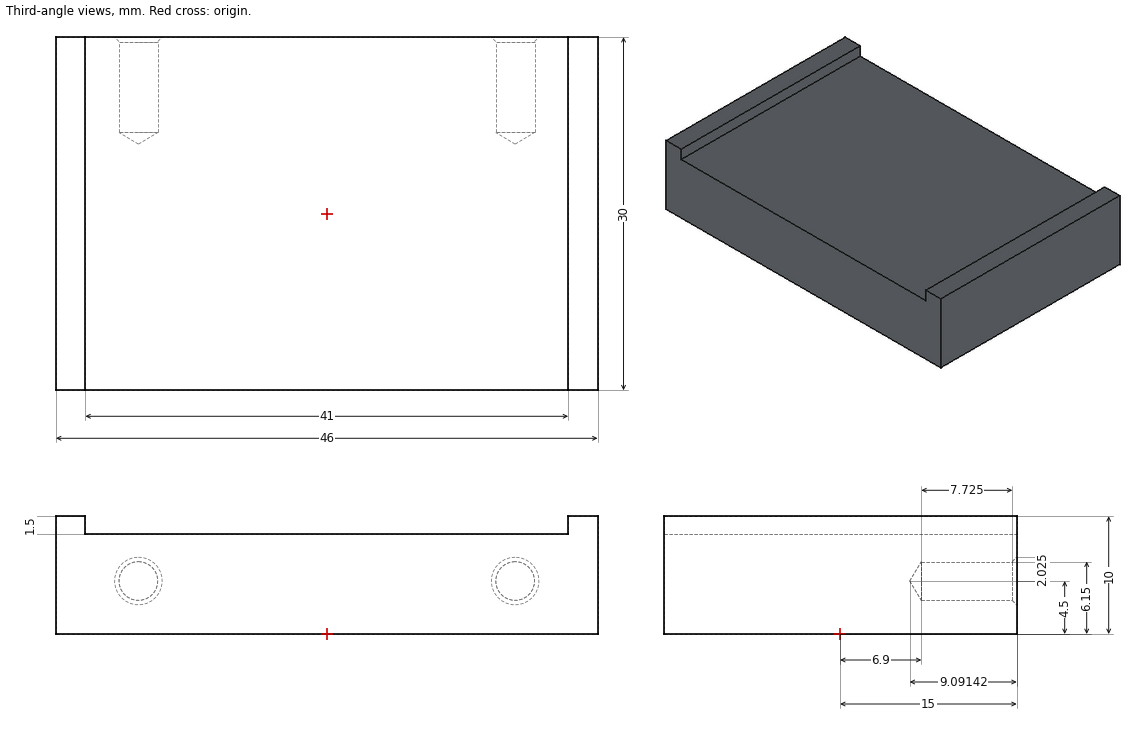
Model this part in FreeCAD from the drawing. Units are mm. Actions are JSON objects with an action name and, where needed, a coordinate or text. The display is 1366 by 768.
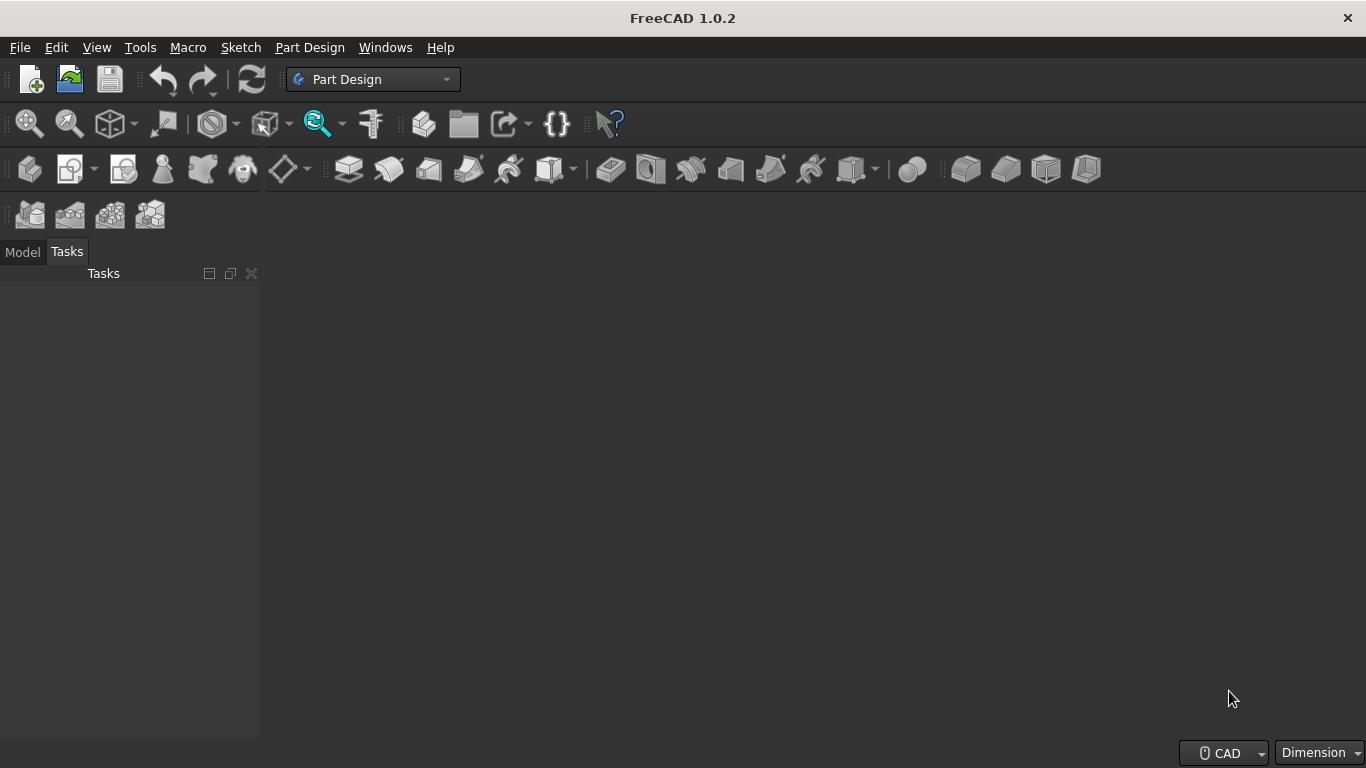
{"action": "left_click", "coordinate": [30, 80]}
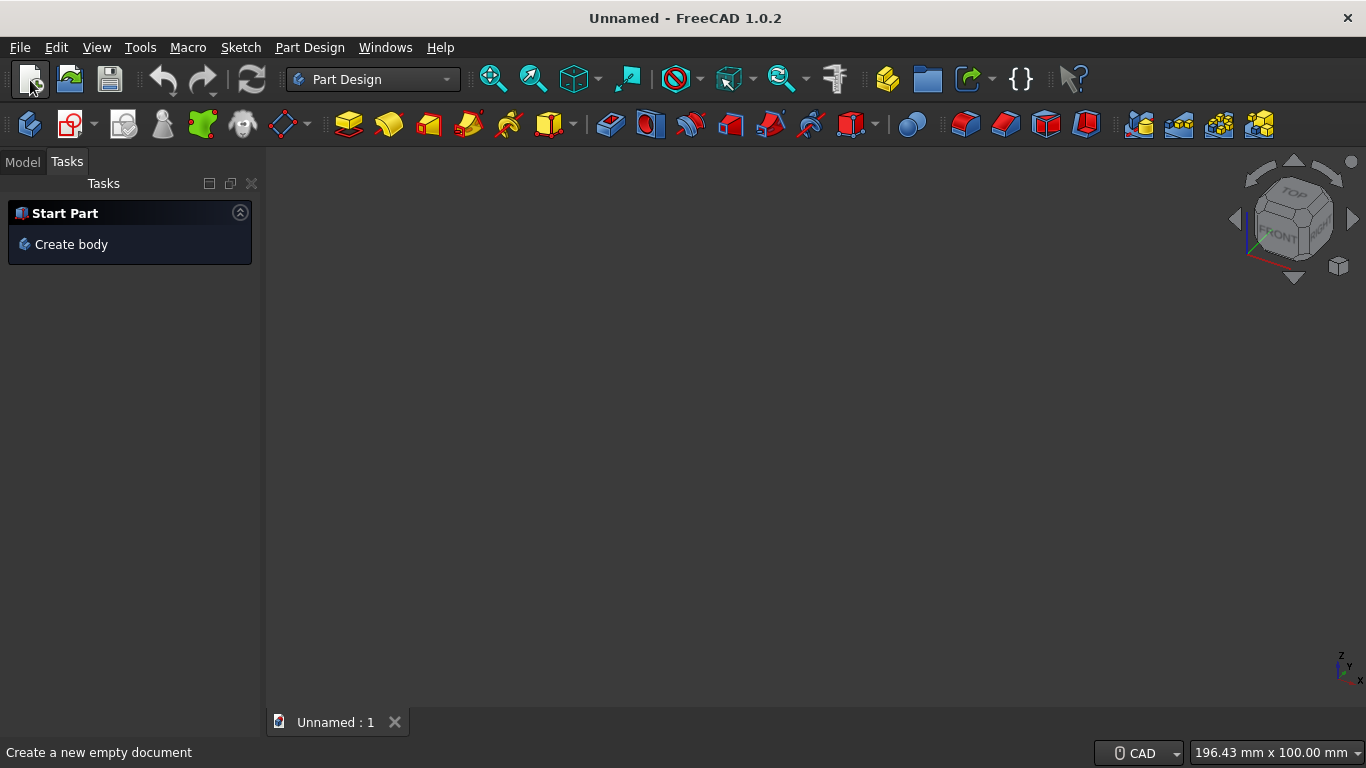
{"action": "left_click", "coordinate": [70, 124]}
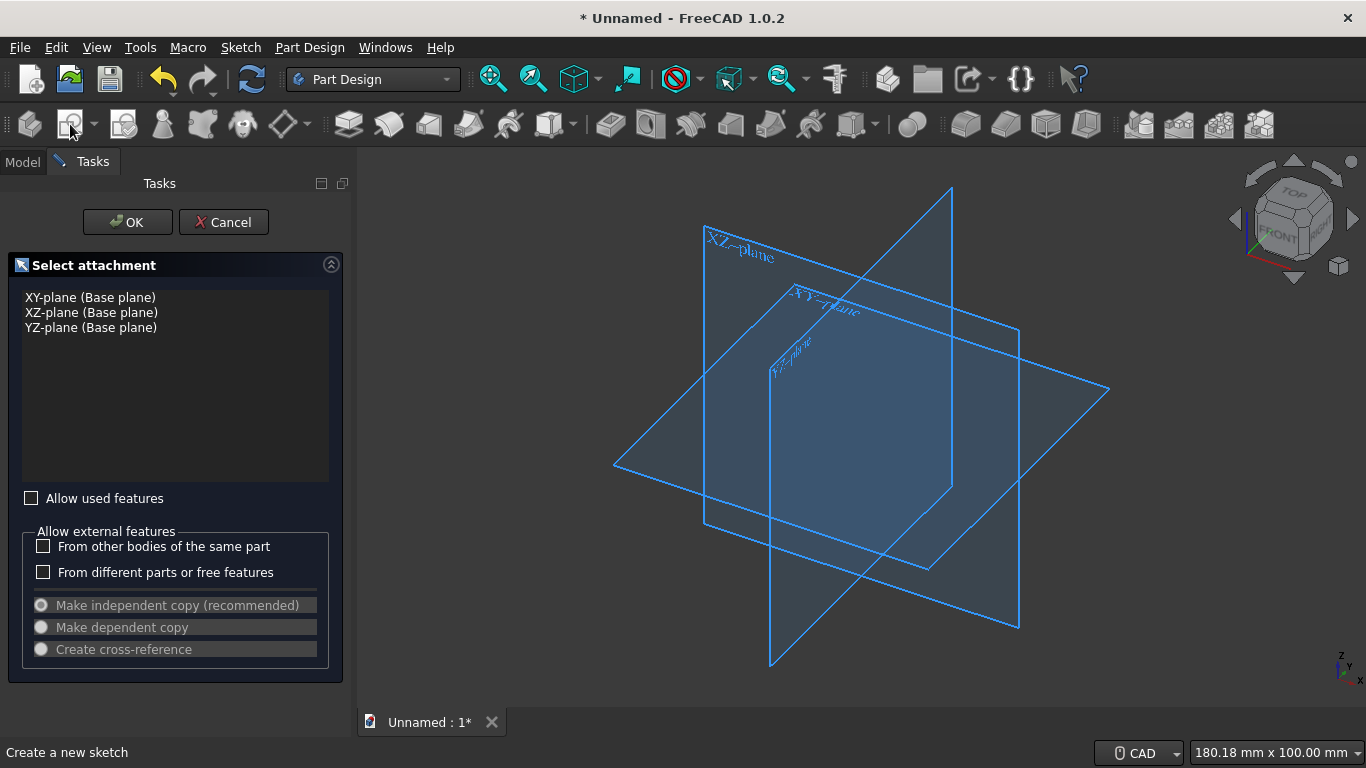
{"action": "left_click", "coordinate": [82, 298]}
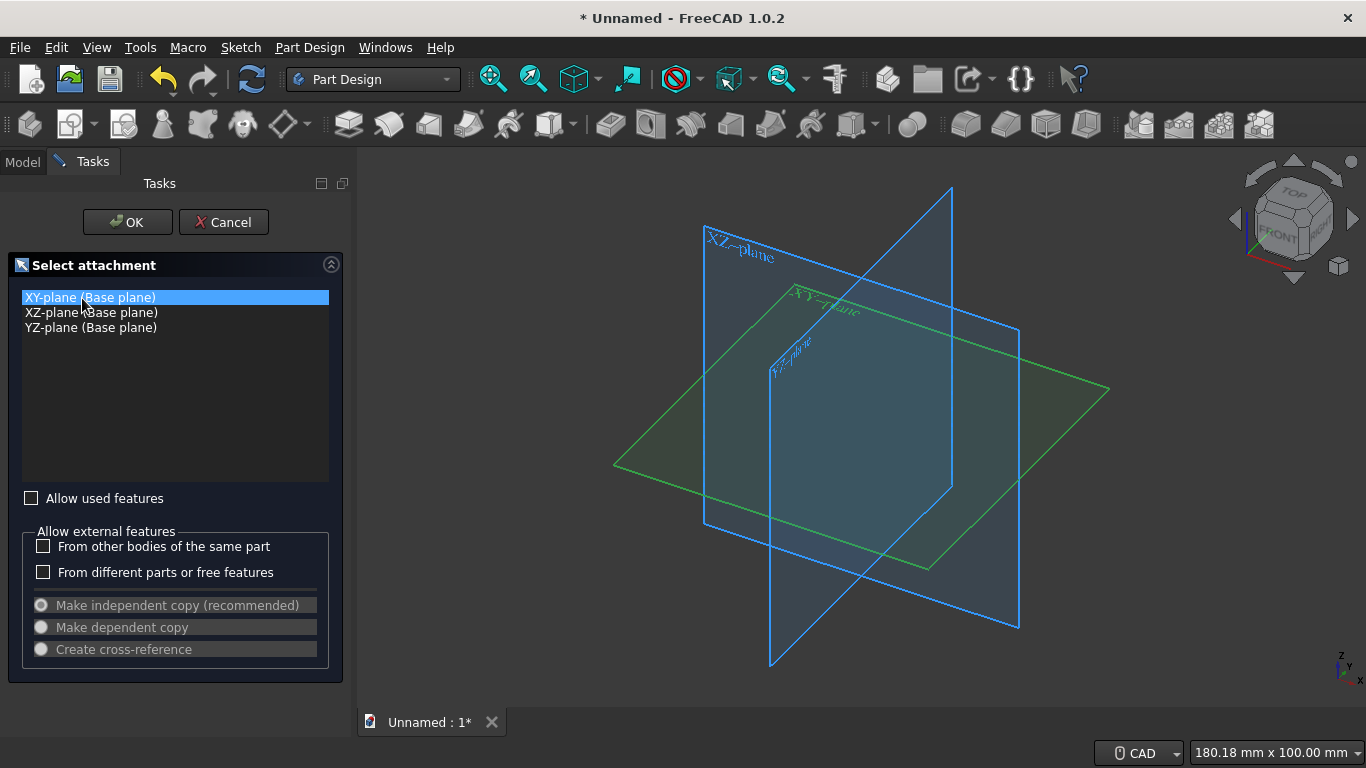
{"action": "left_click", "coordinate": [128, 222]}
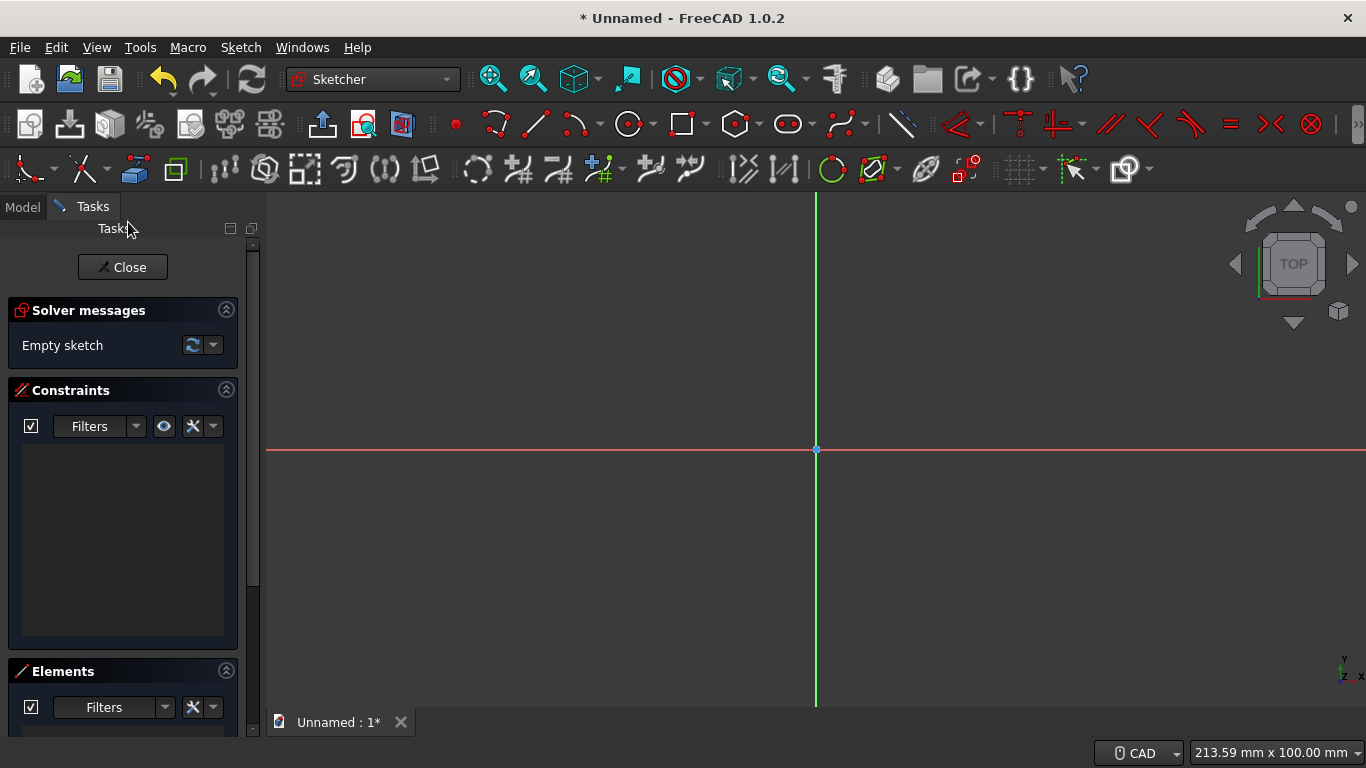
{"action": "scroll", "coordinate": [872, 450], "scroll_direction": "up", "scroll_amount": 4}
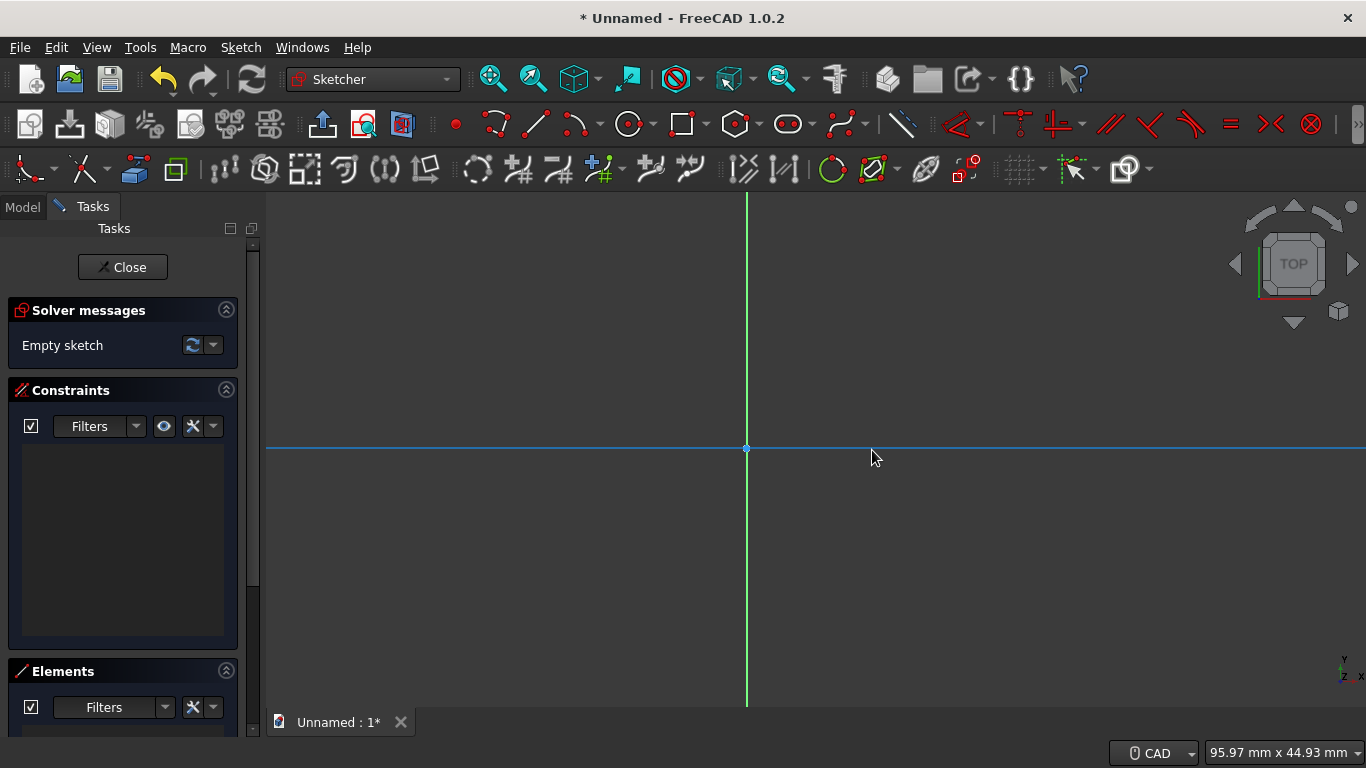
{"action": "left_click", "coordinate": [708, 124]}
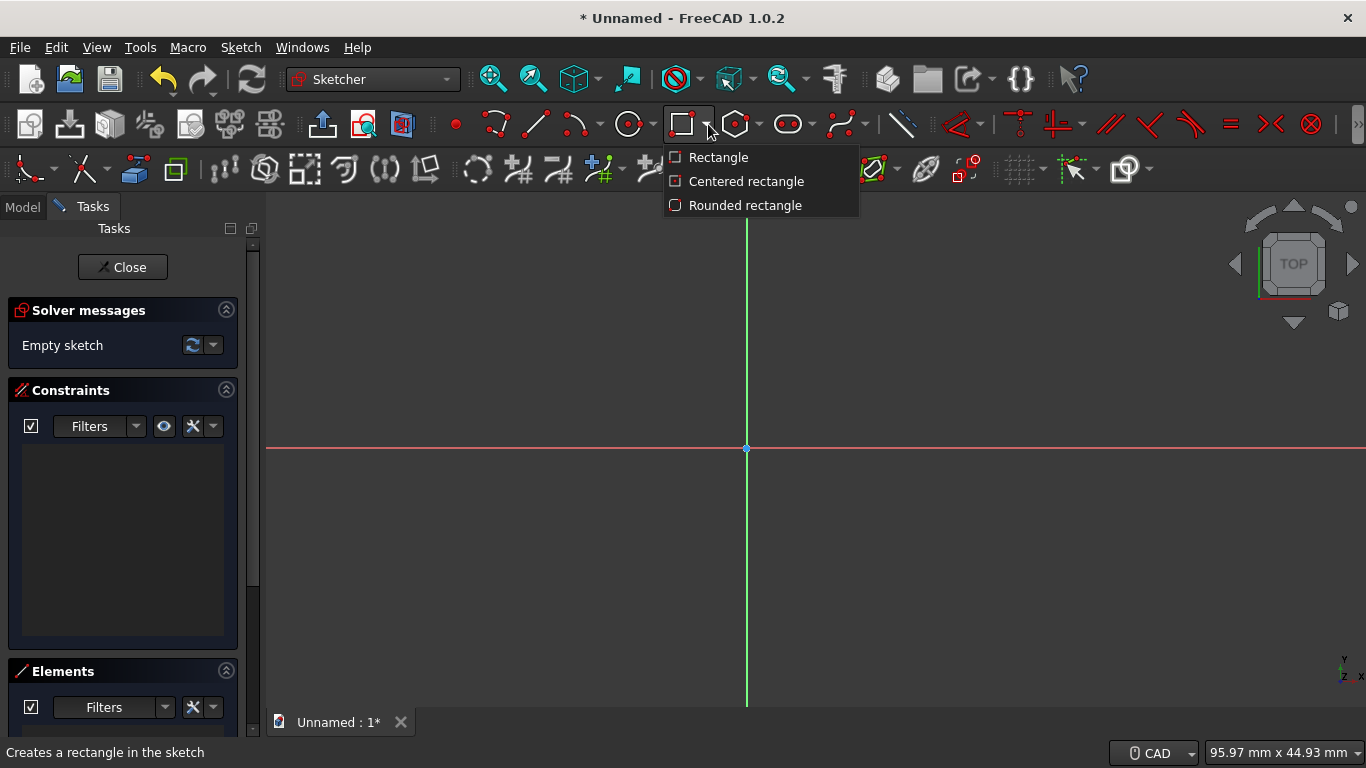
{"action": "left_click", "coordinate": [762, 181]}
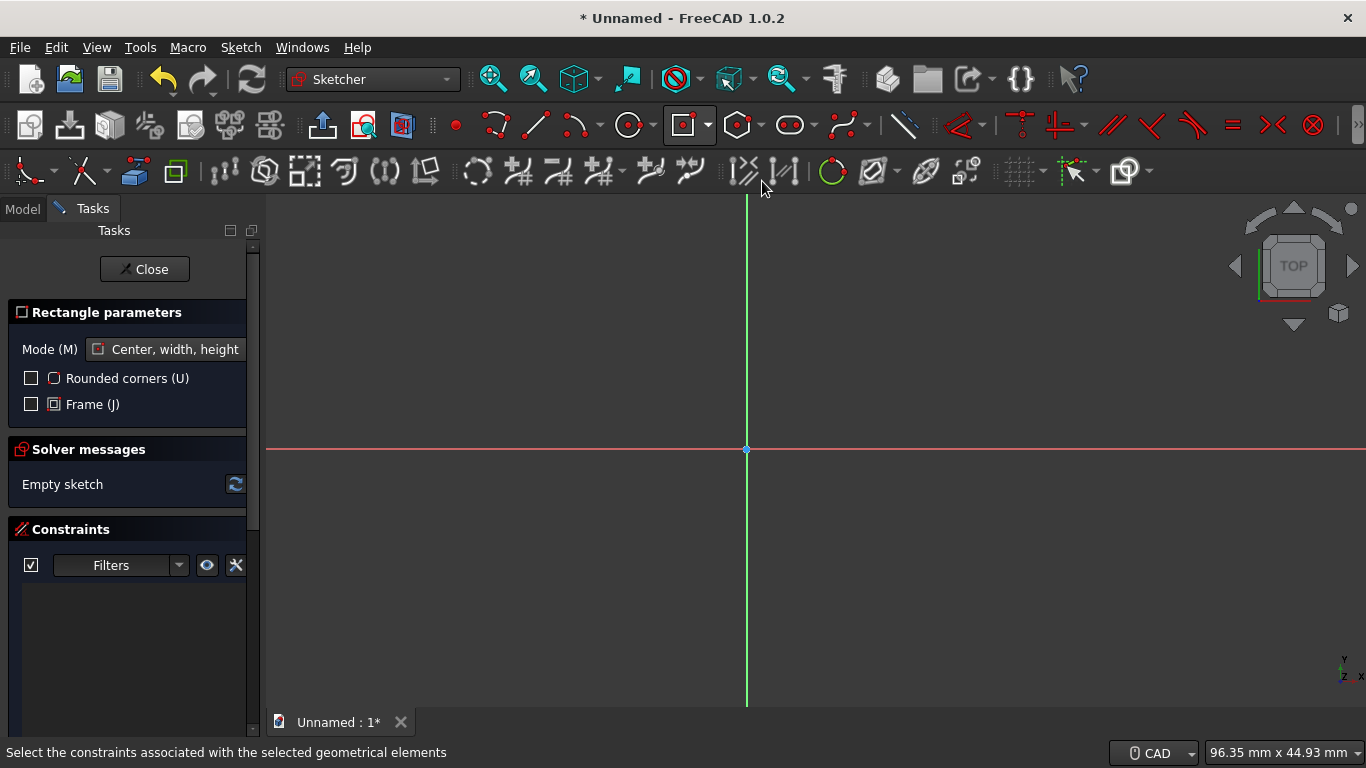
{"action": "left_click", "coordinate": [747, 449]}
{"action": "mouse_move", "coordinate": [1010, 278]}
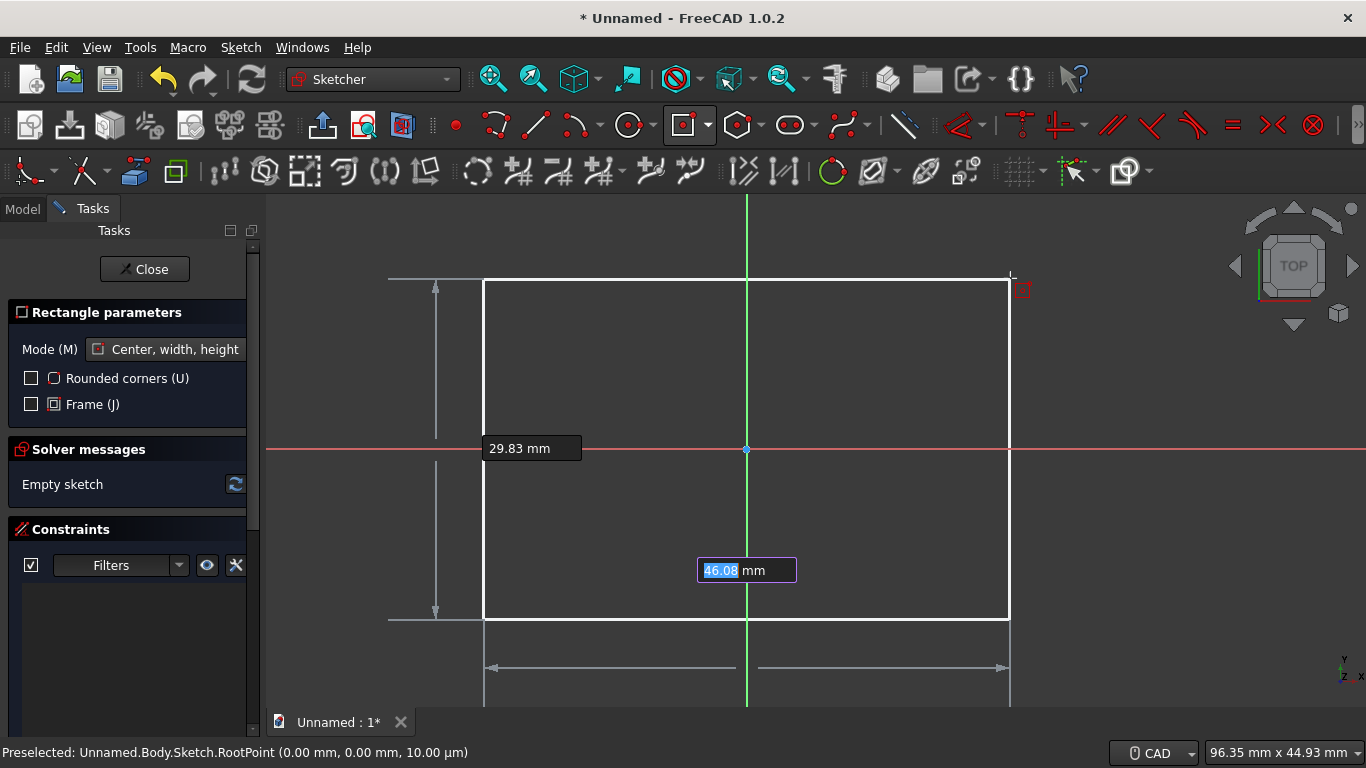
{"action": "type", "text": "46"}
{"action": "key", "text": "Tab"}
{"action": "type", "text": "30"}
{"action": "key", "text": "Return"}
{"action": "key", "text": "Escape"}